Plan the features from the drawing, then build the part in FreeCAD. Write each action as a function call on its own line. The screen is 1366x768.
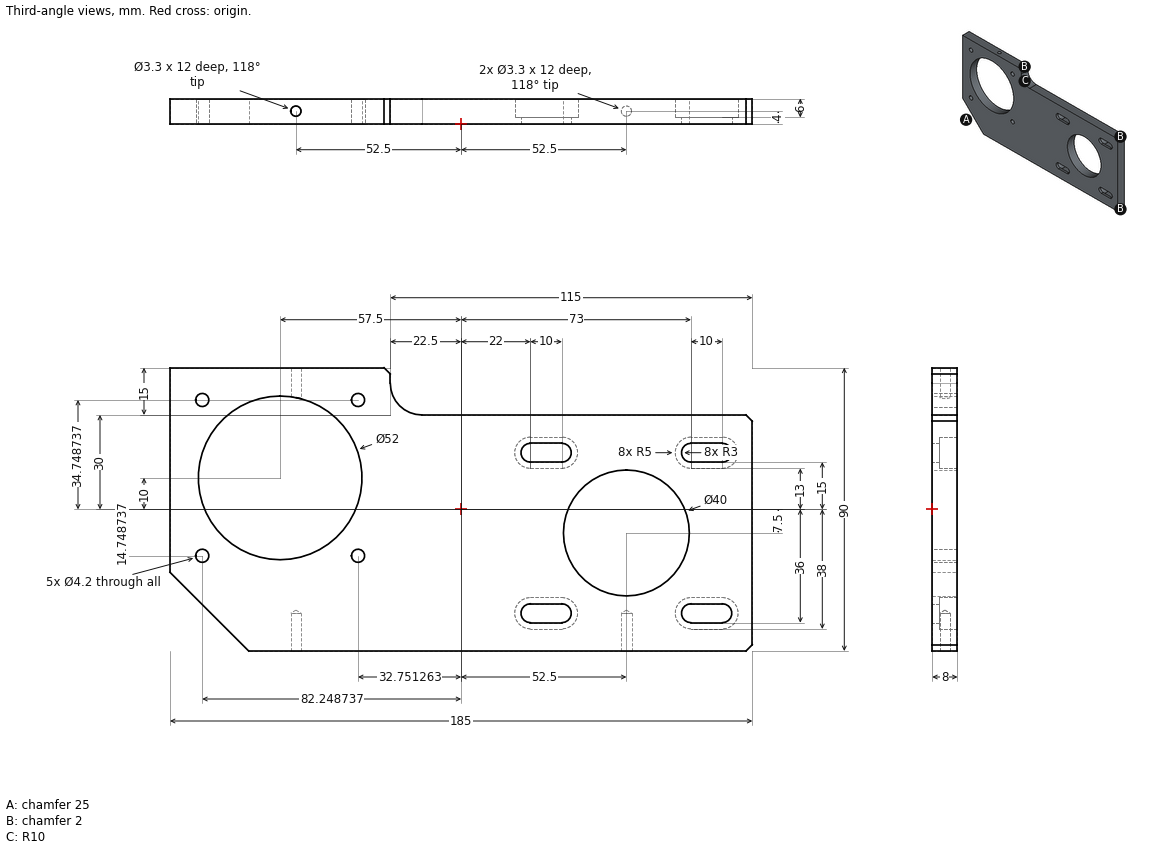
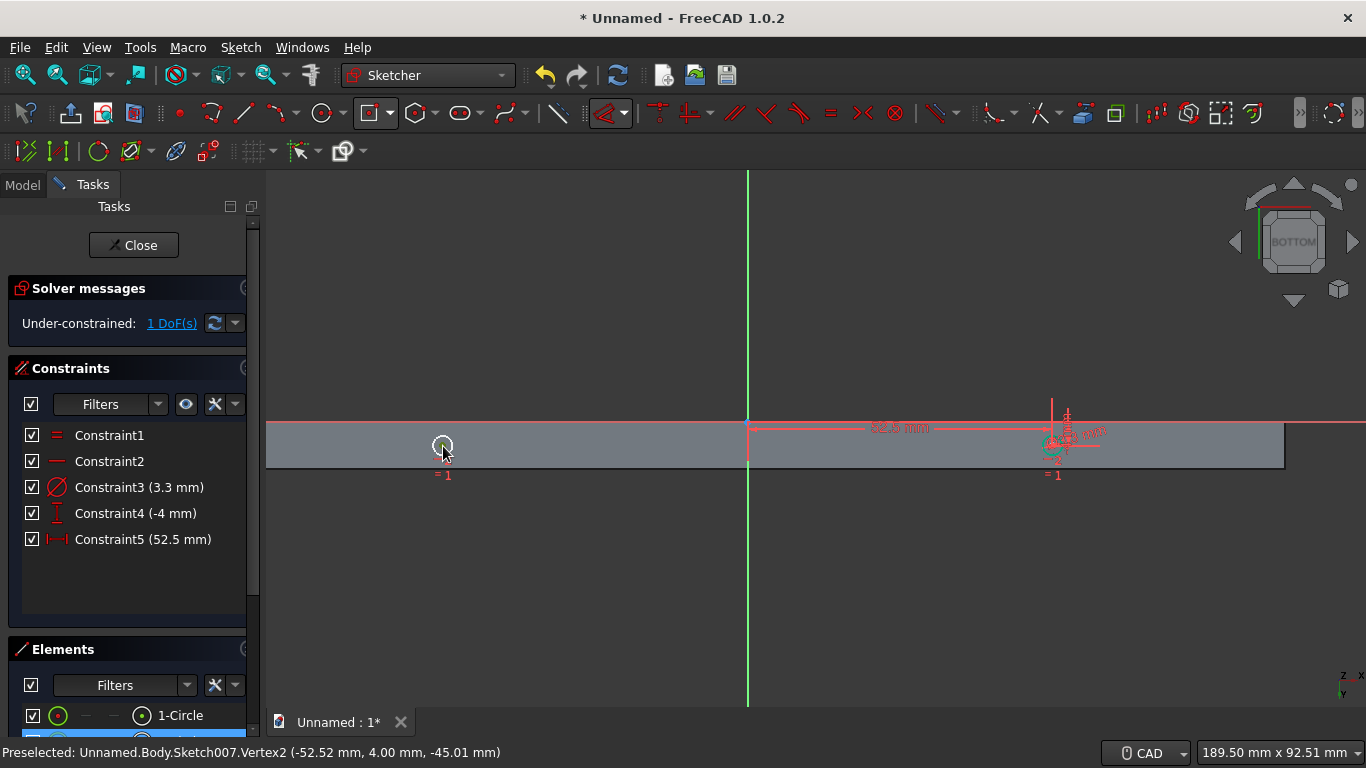
key(l)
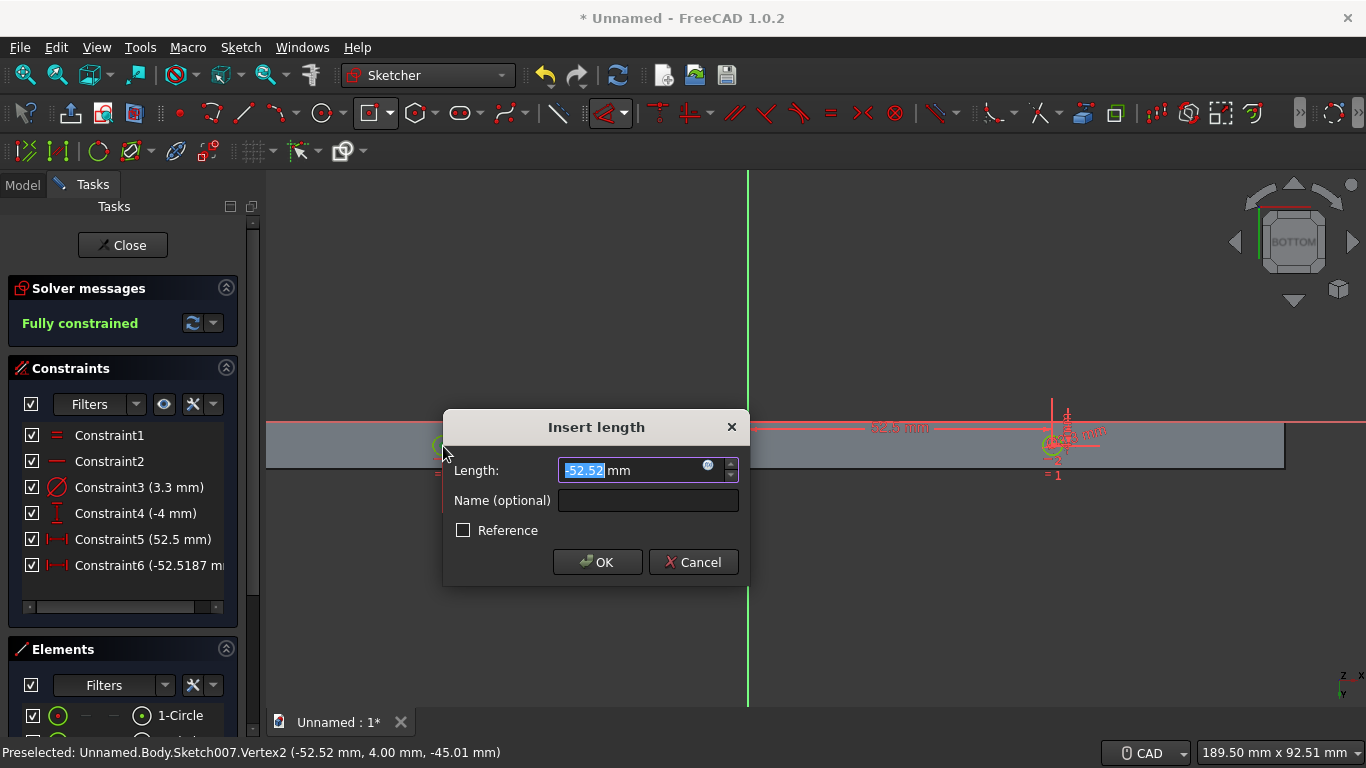
text(-52.5)
key(Return)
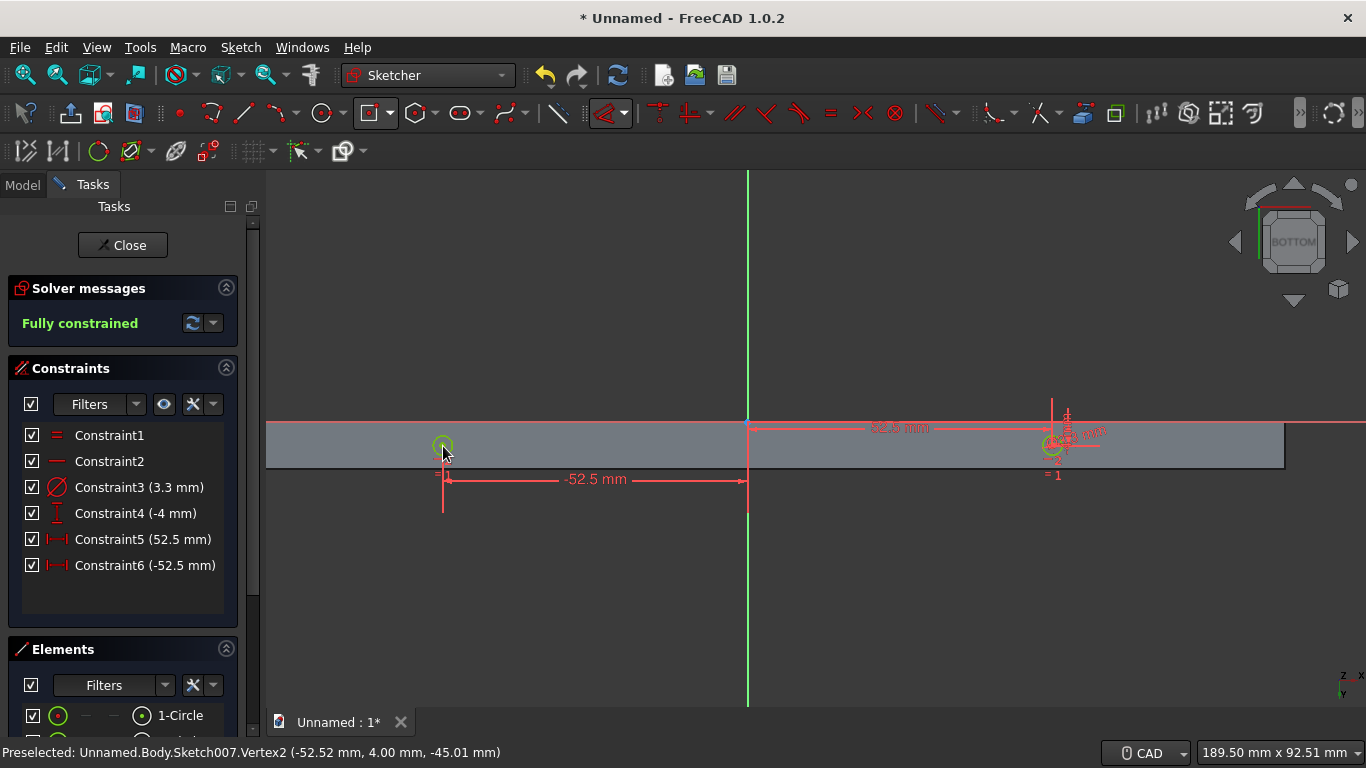
click(123, 245)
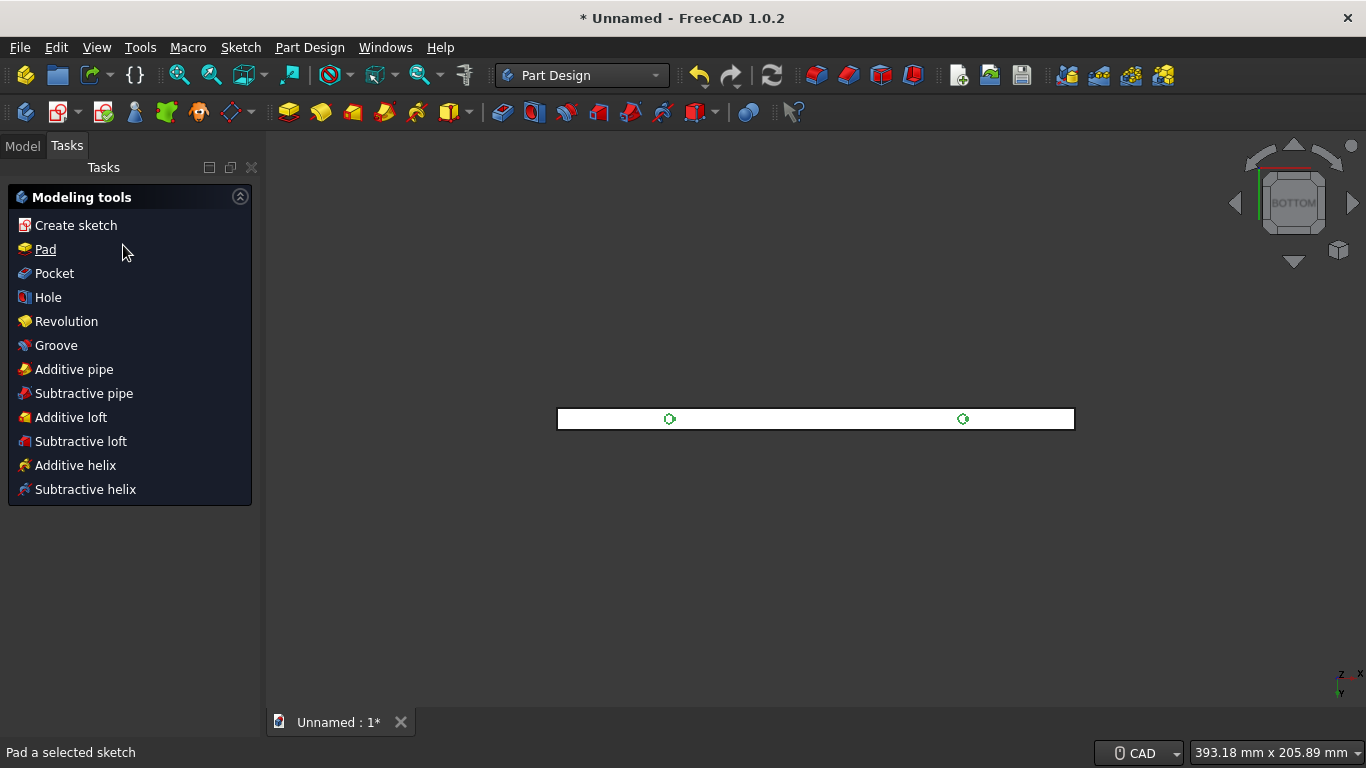
click(536, 112)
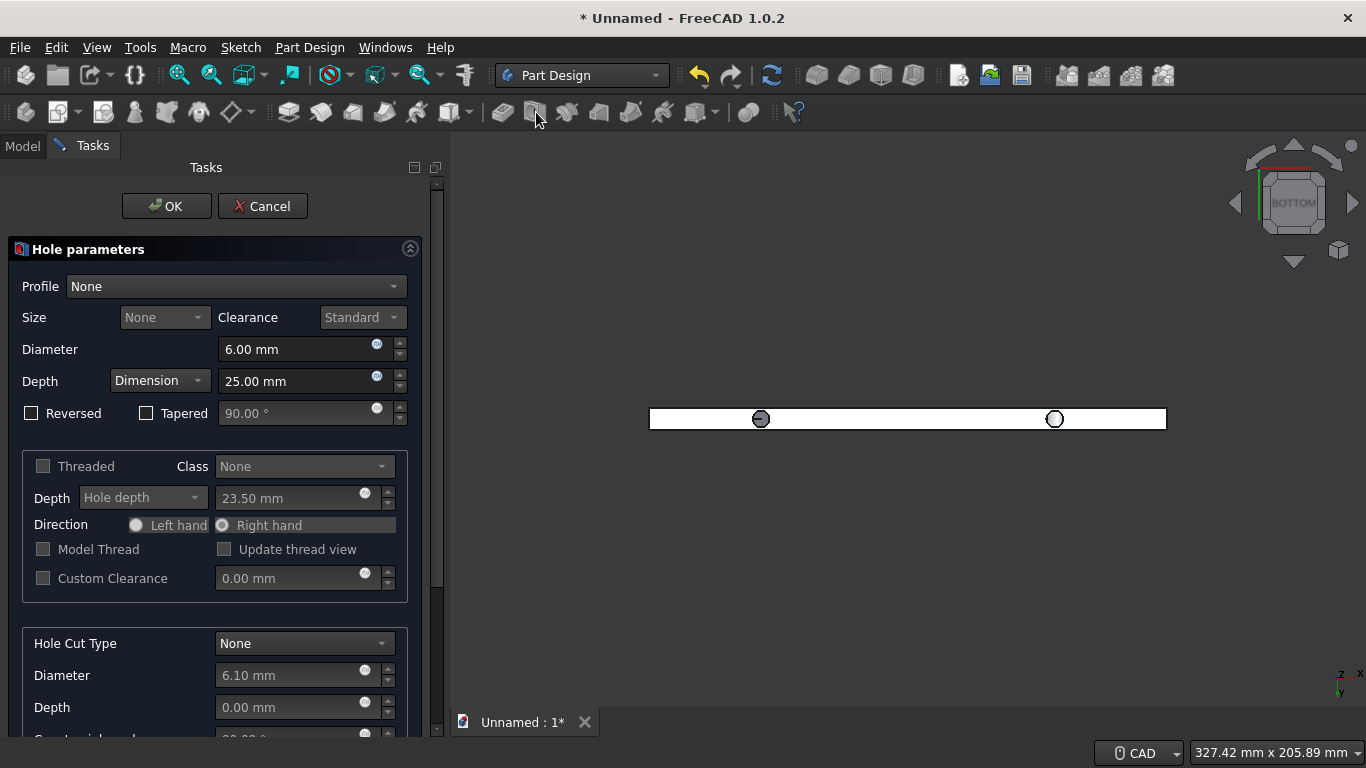
triple_click(305, 349)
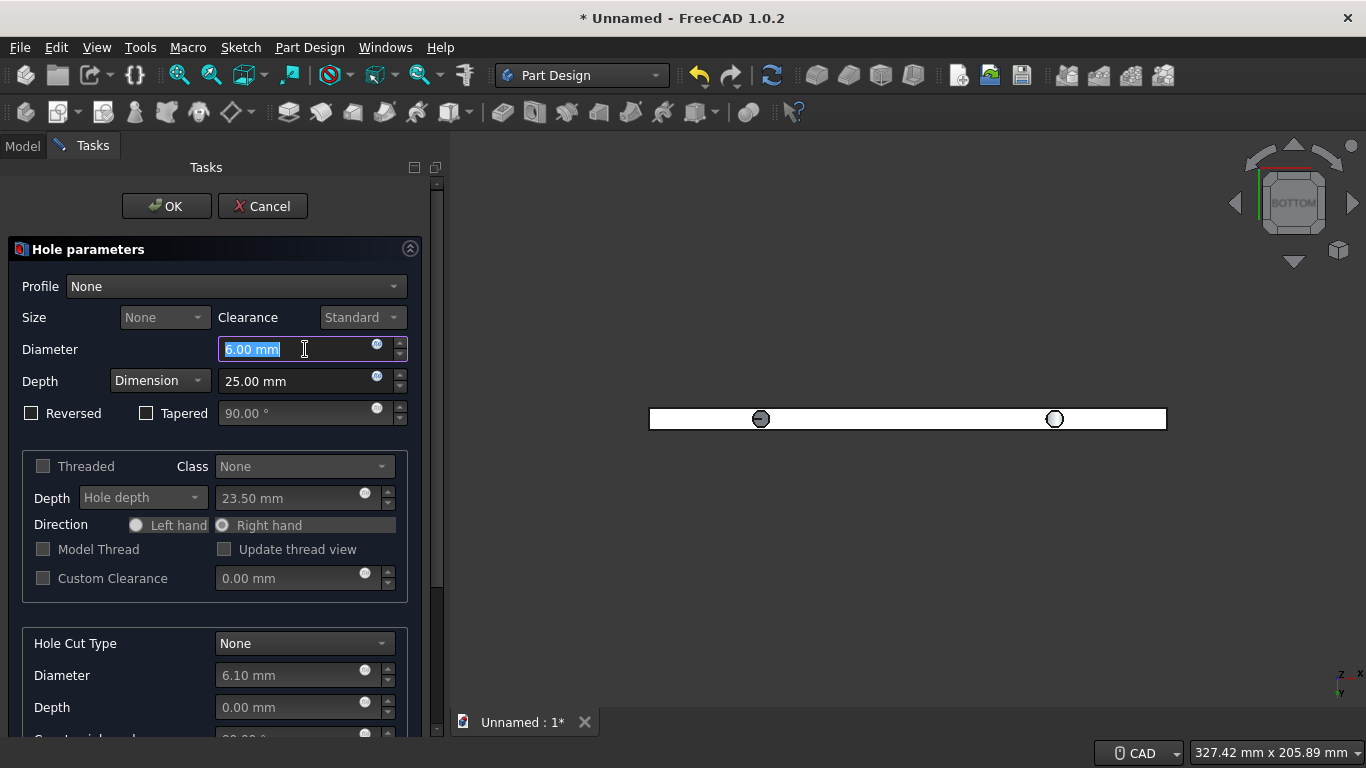
text(3.3)
key(Tab)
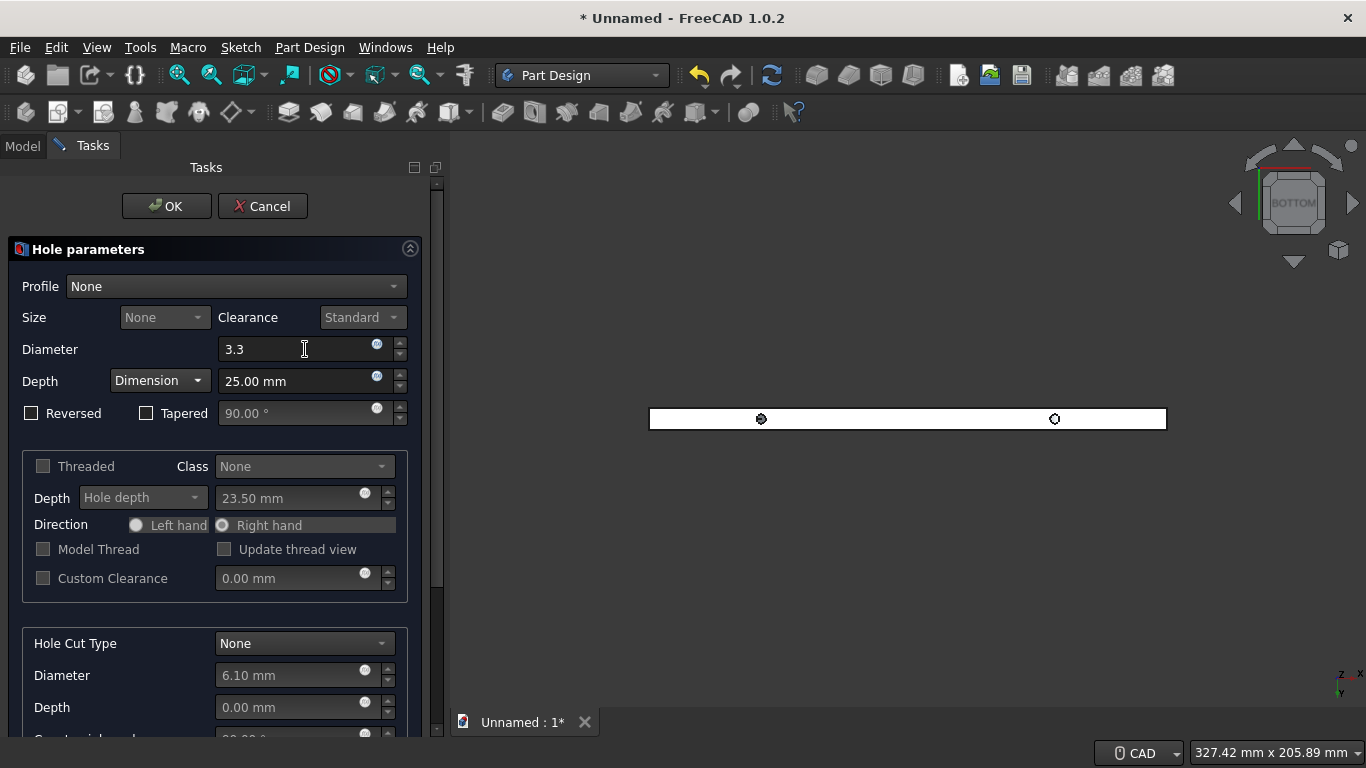
triple_click(305, 381)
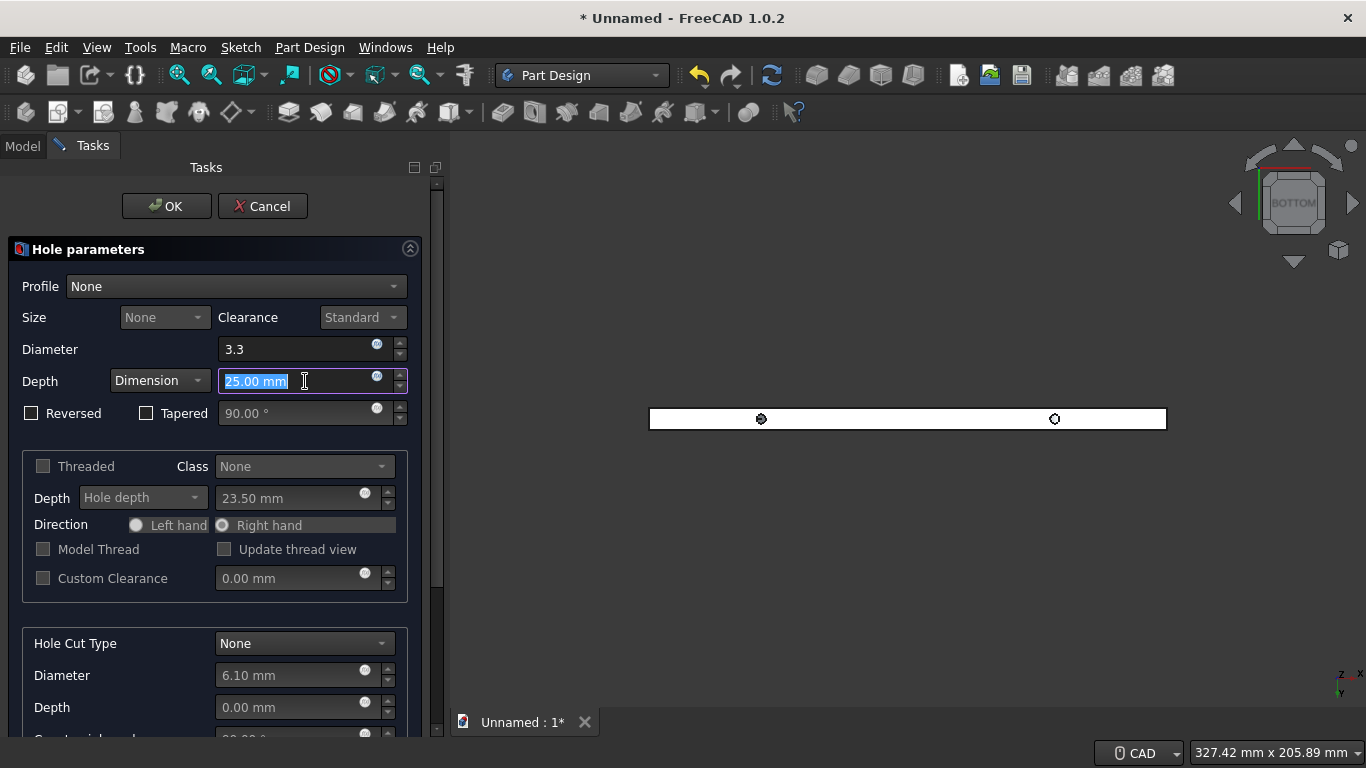
text(12)
key(Tab)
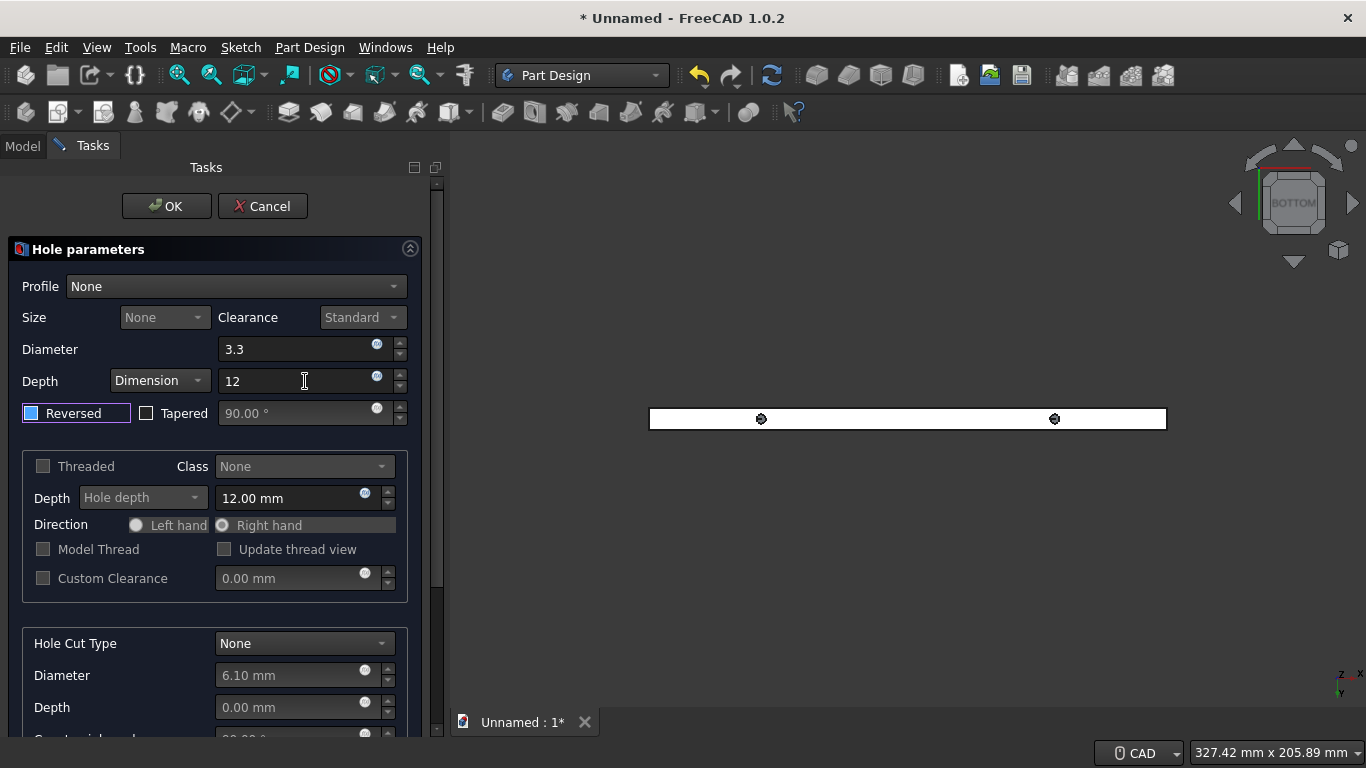
click(167, 206)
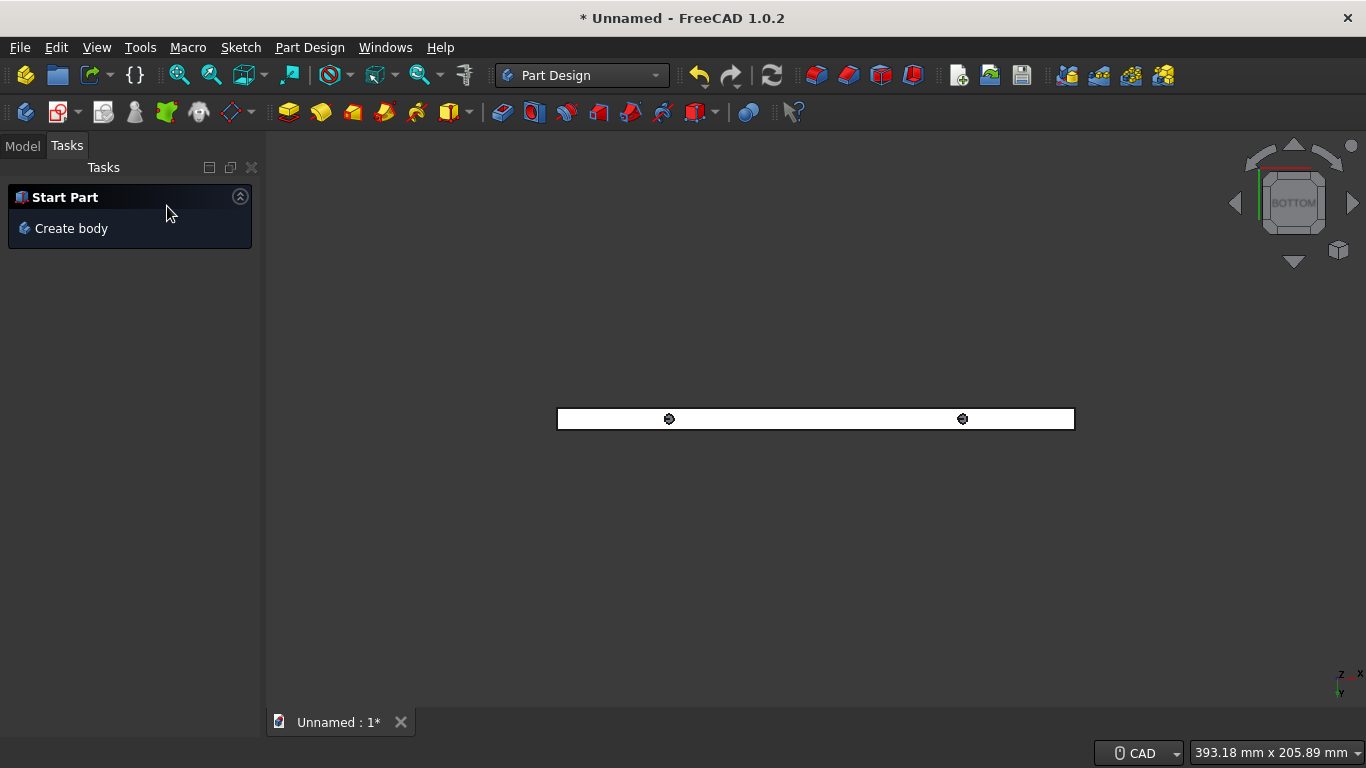
key(0)